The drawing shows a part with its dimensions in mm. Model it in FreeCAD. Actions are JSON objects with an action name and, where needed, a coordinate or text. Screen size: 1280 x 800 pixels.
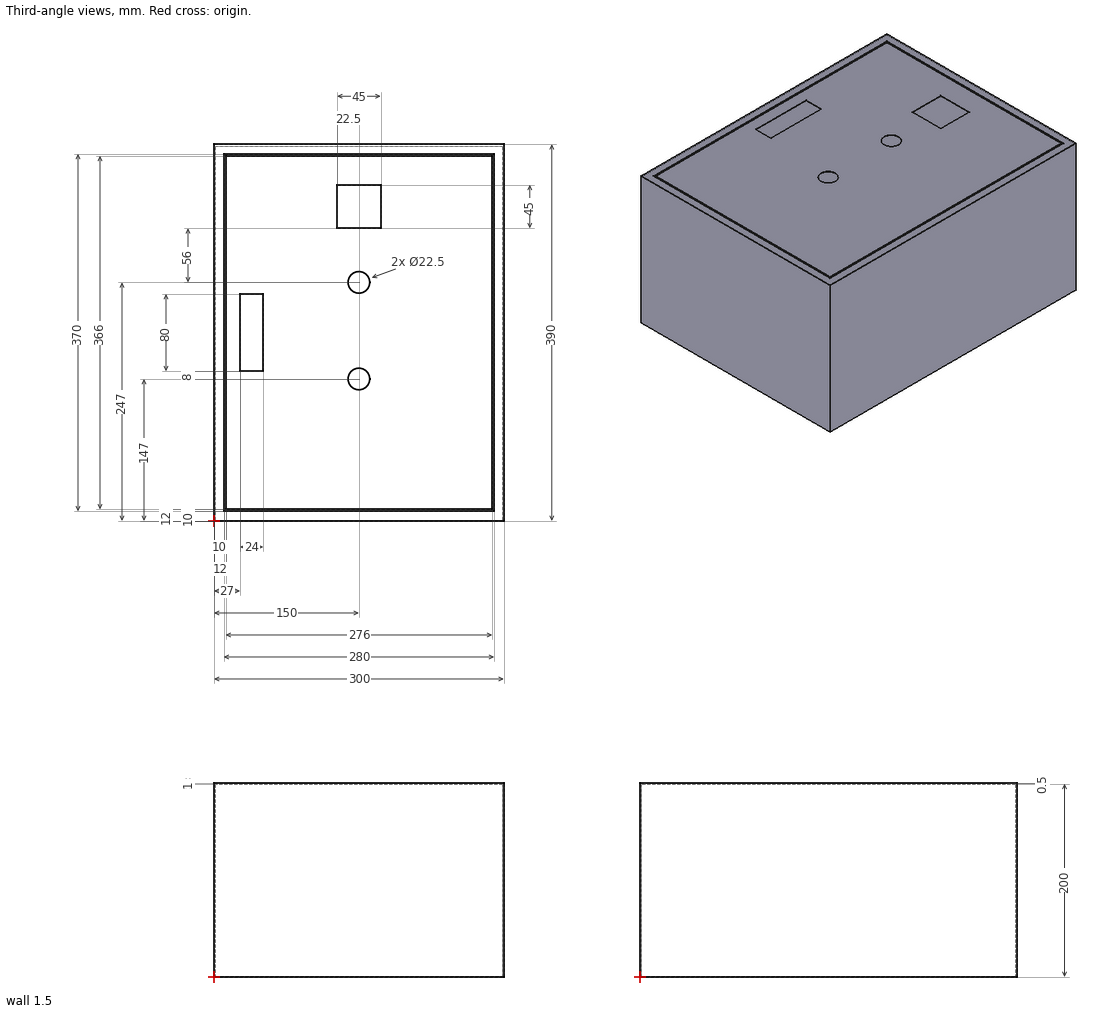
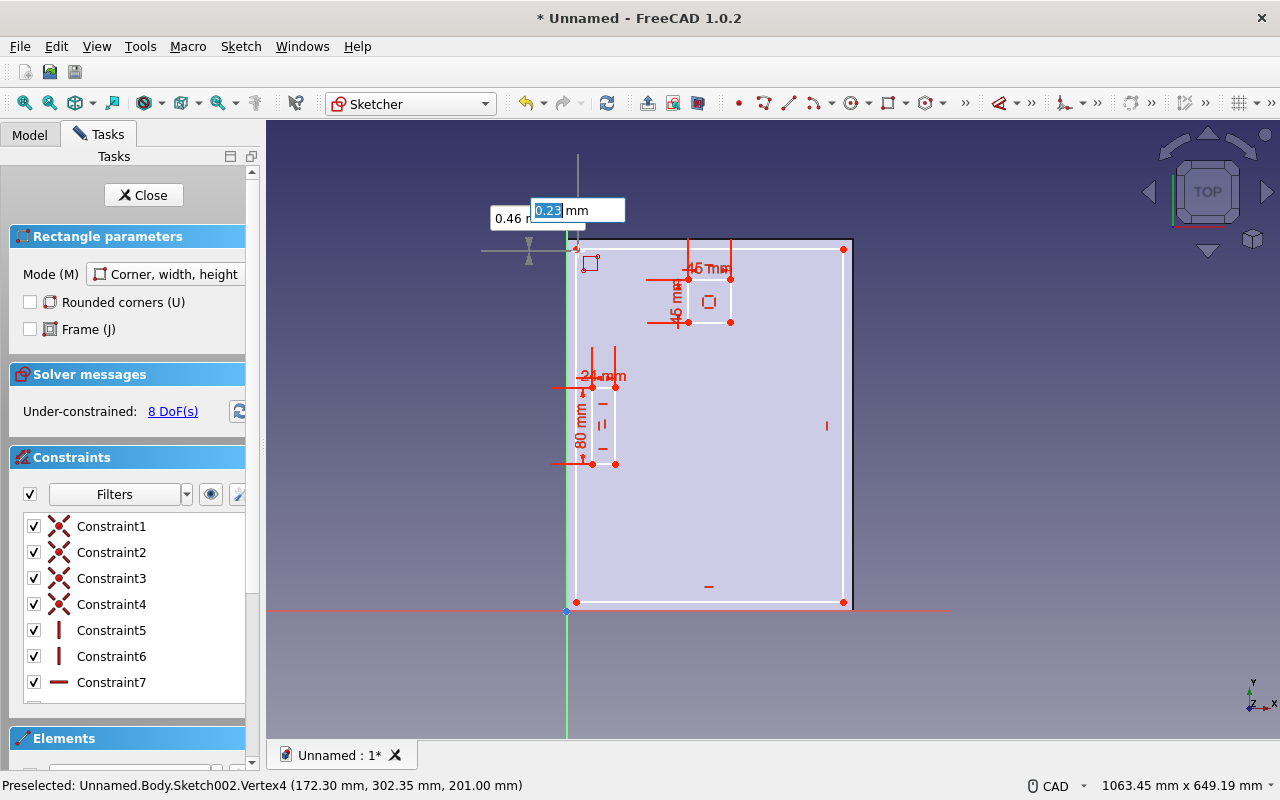
{"action": "scroll", "coordinate": [841, 600], "scroll_direction": "up", "scroll_amount": 11}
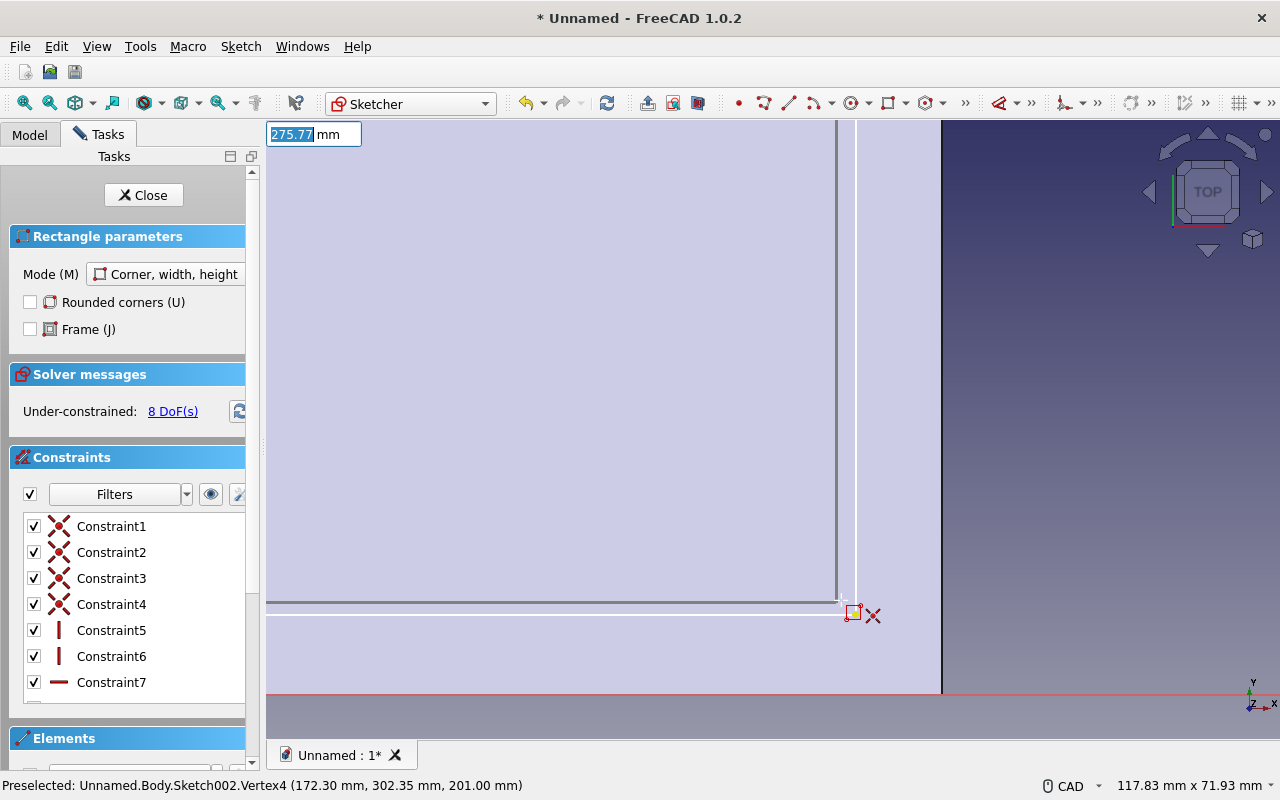
{"action": "left_click", "coordinate": [838, 592]}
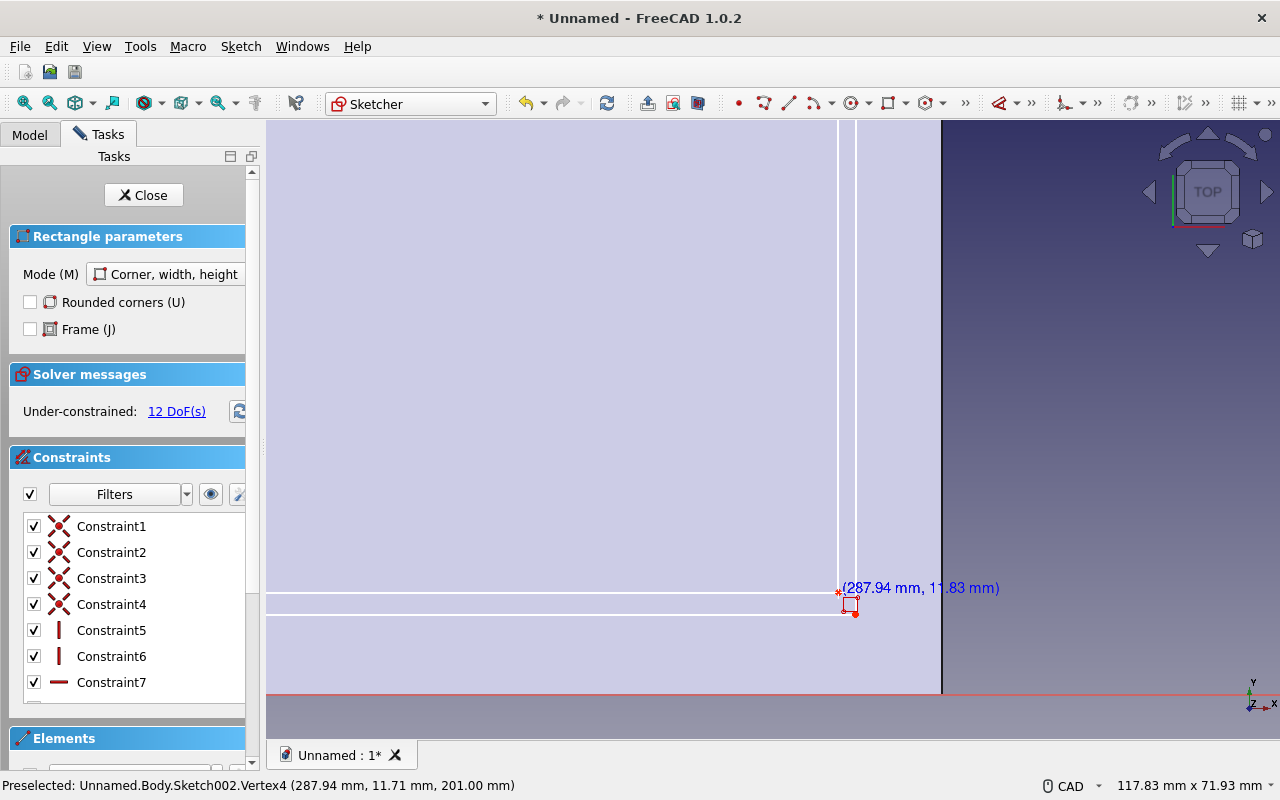
{"action": "left_click", "coordinate": [850, 104]}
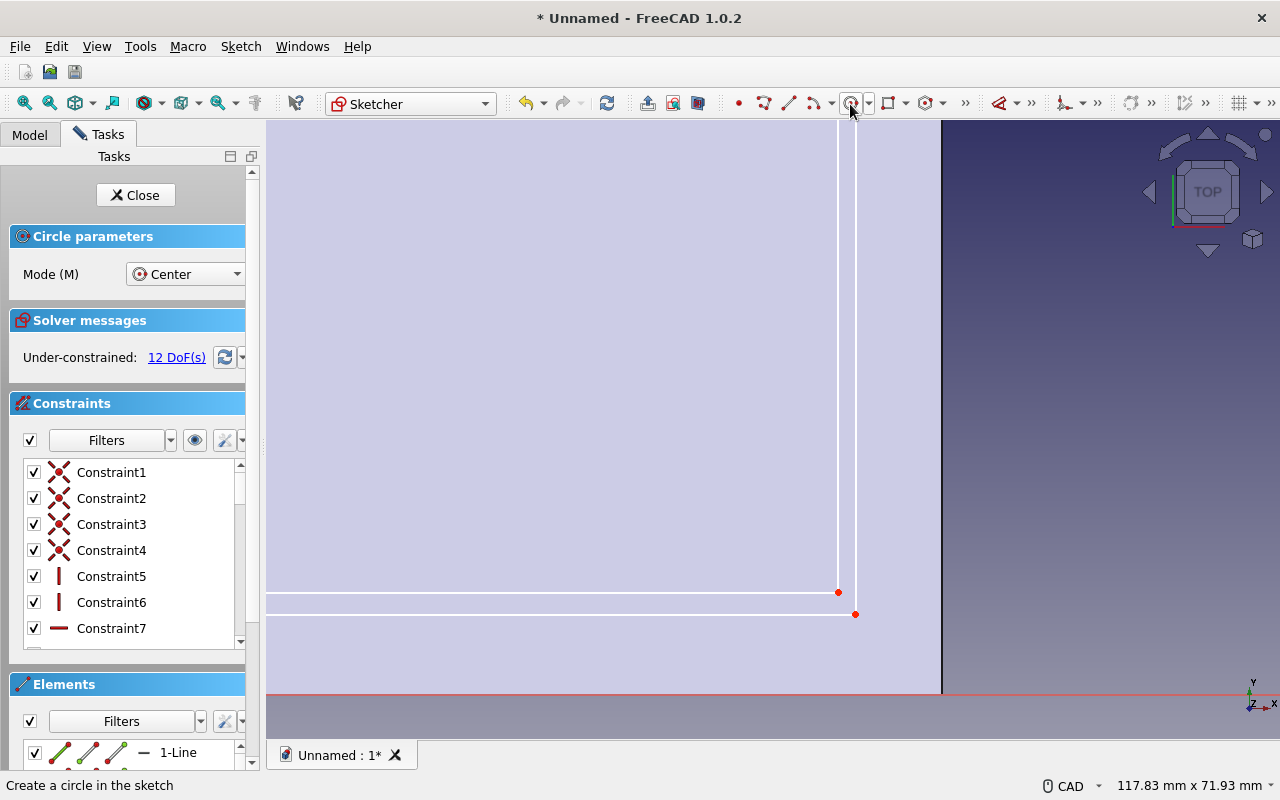
{"action": "scroll", "coordinate": [841, 600], "scroll_direction": "down", "scroll_amount": 11}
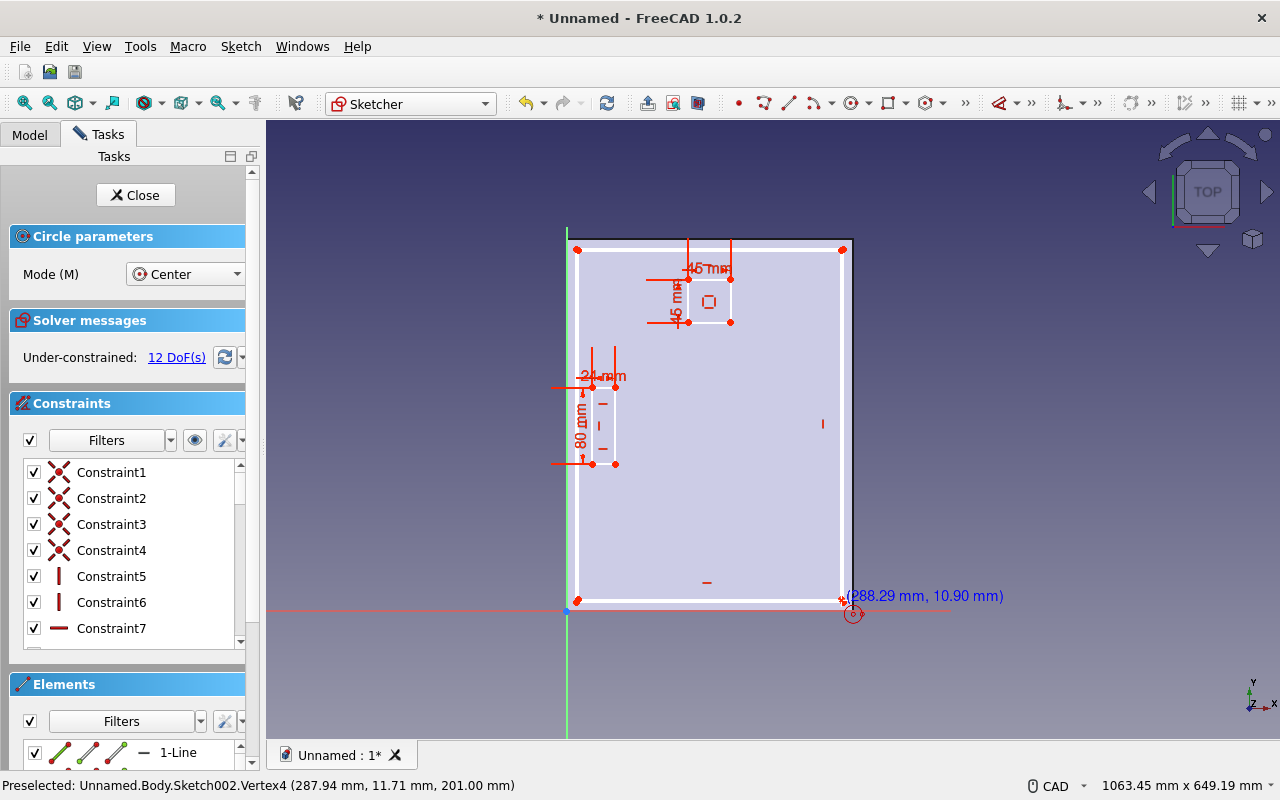
{"action": "scroll", "coordinate": [710, 376], "scroll_direction": "up", "scroll_amount": 4}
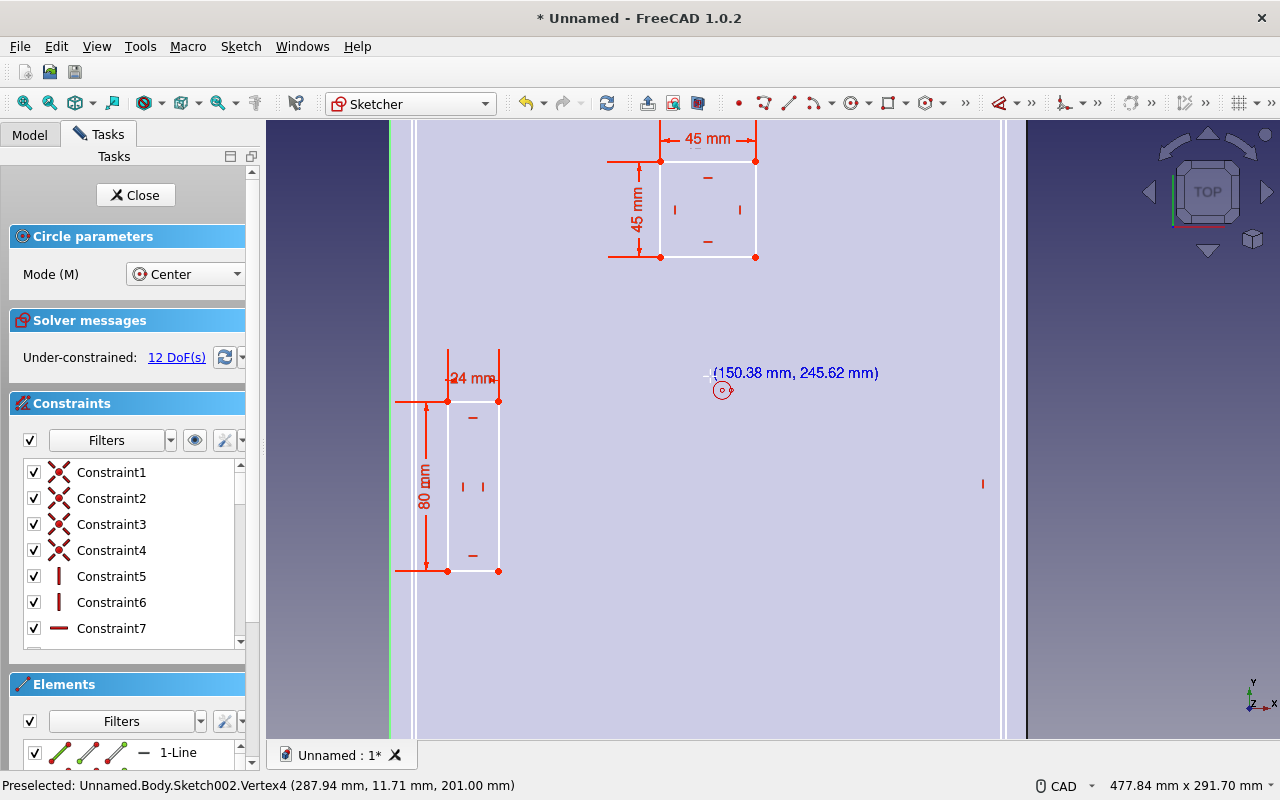
{"action": "left_click", "coordinate": [709, 375]}
{"action": "mouse_move", "coordinate": [726, 358]}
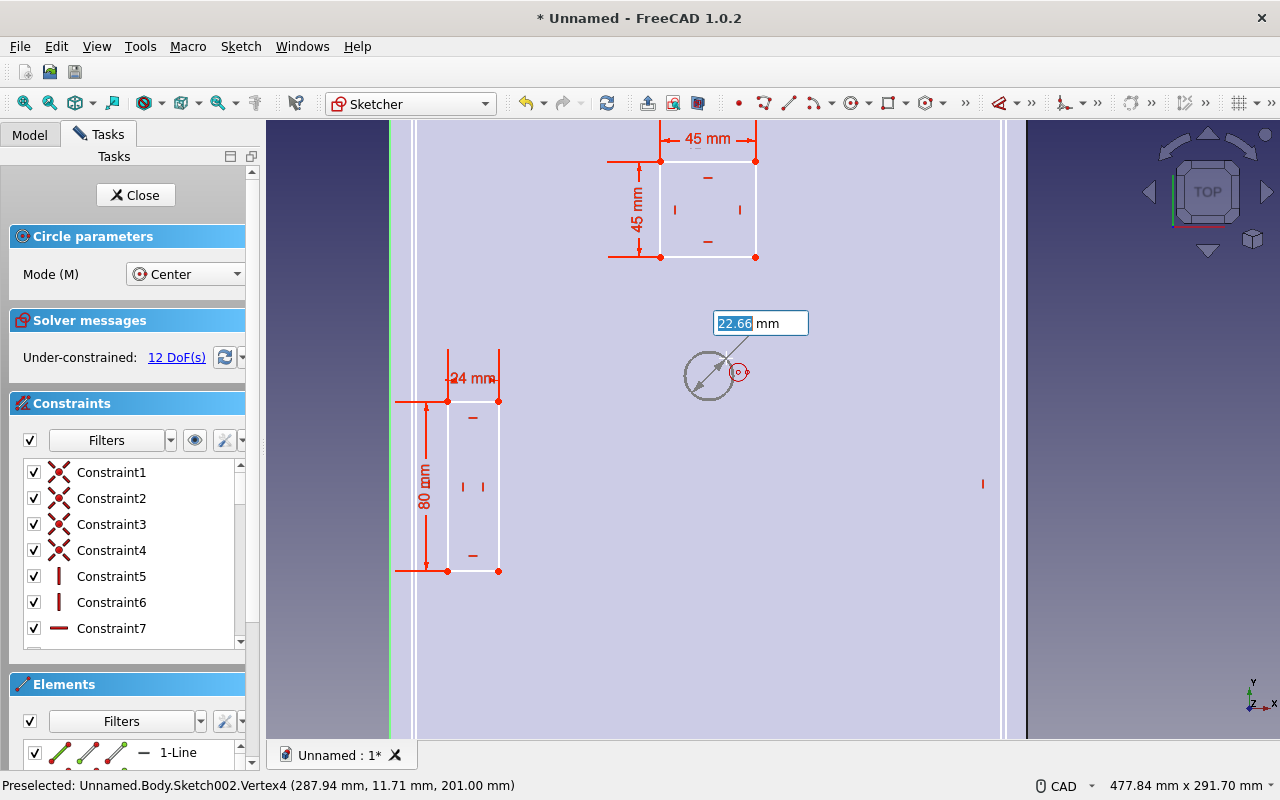
{"action": "type", "text": "22.5"}
{"action": "key", "text": "Return"}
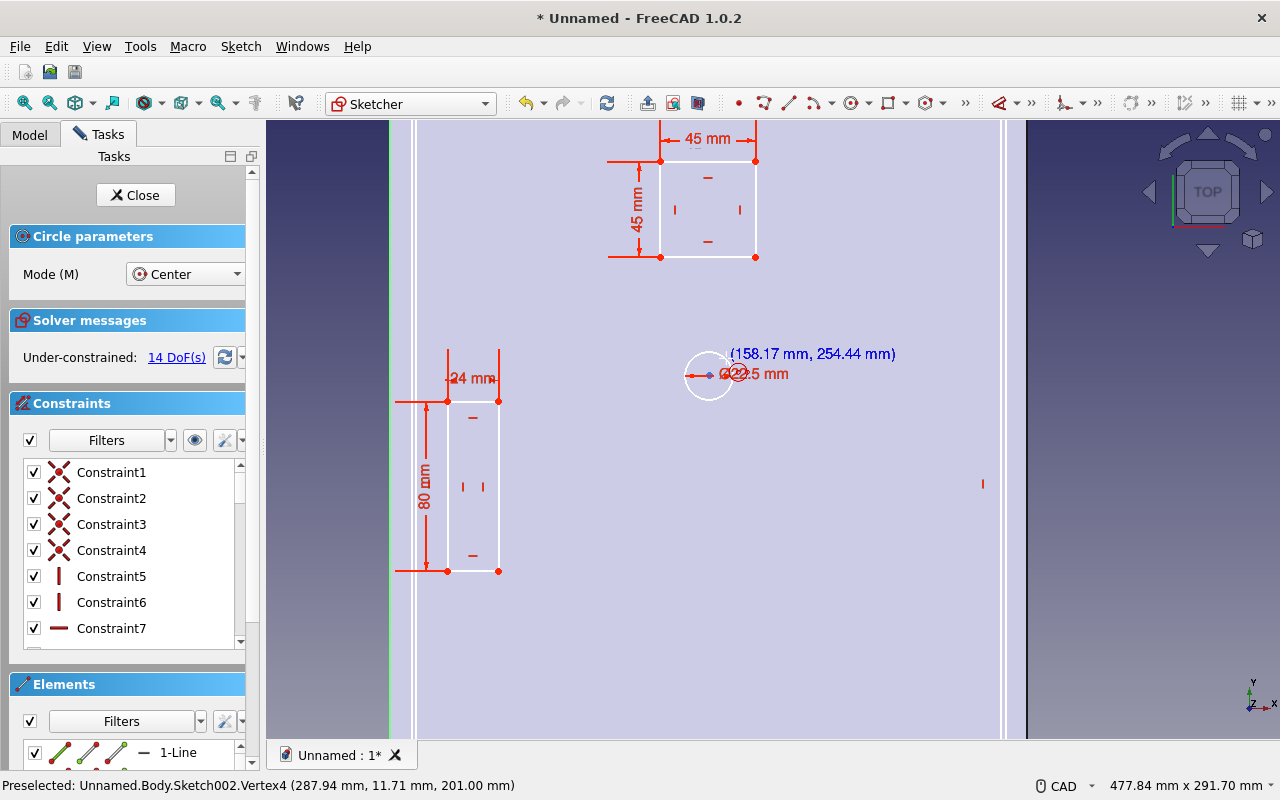
{"action": "left_click", "coordinate": [709, 587]}
{"action": "mouse_move", "coordinate": [726, 570]}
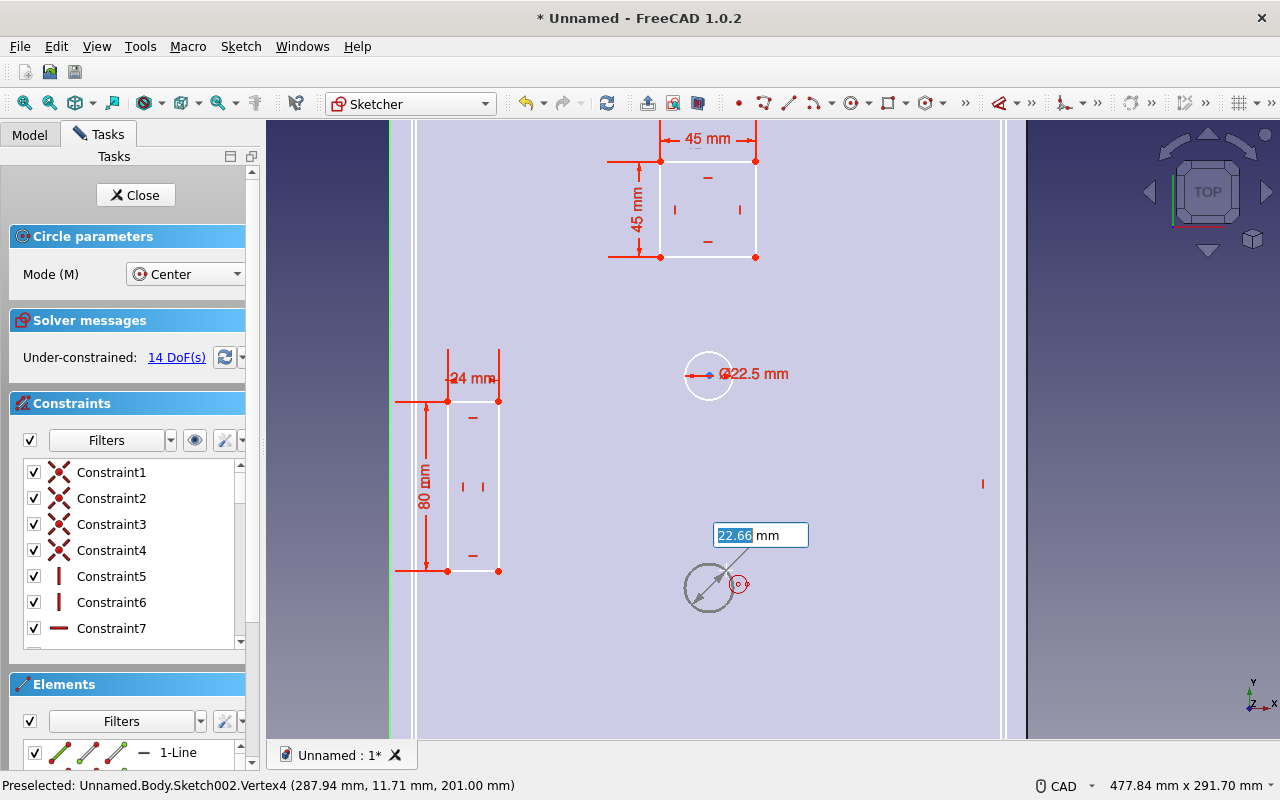
{"action": "type", "text": "22.5"}
{"action": "key", "text": "Return"}
{"action": "key", "text": "Escape"}